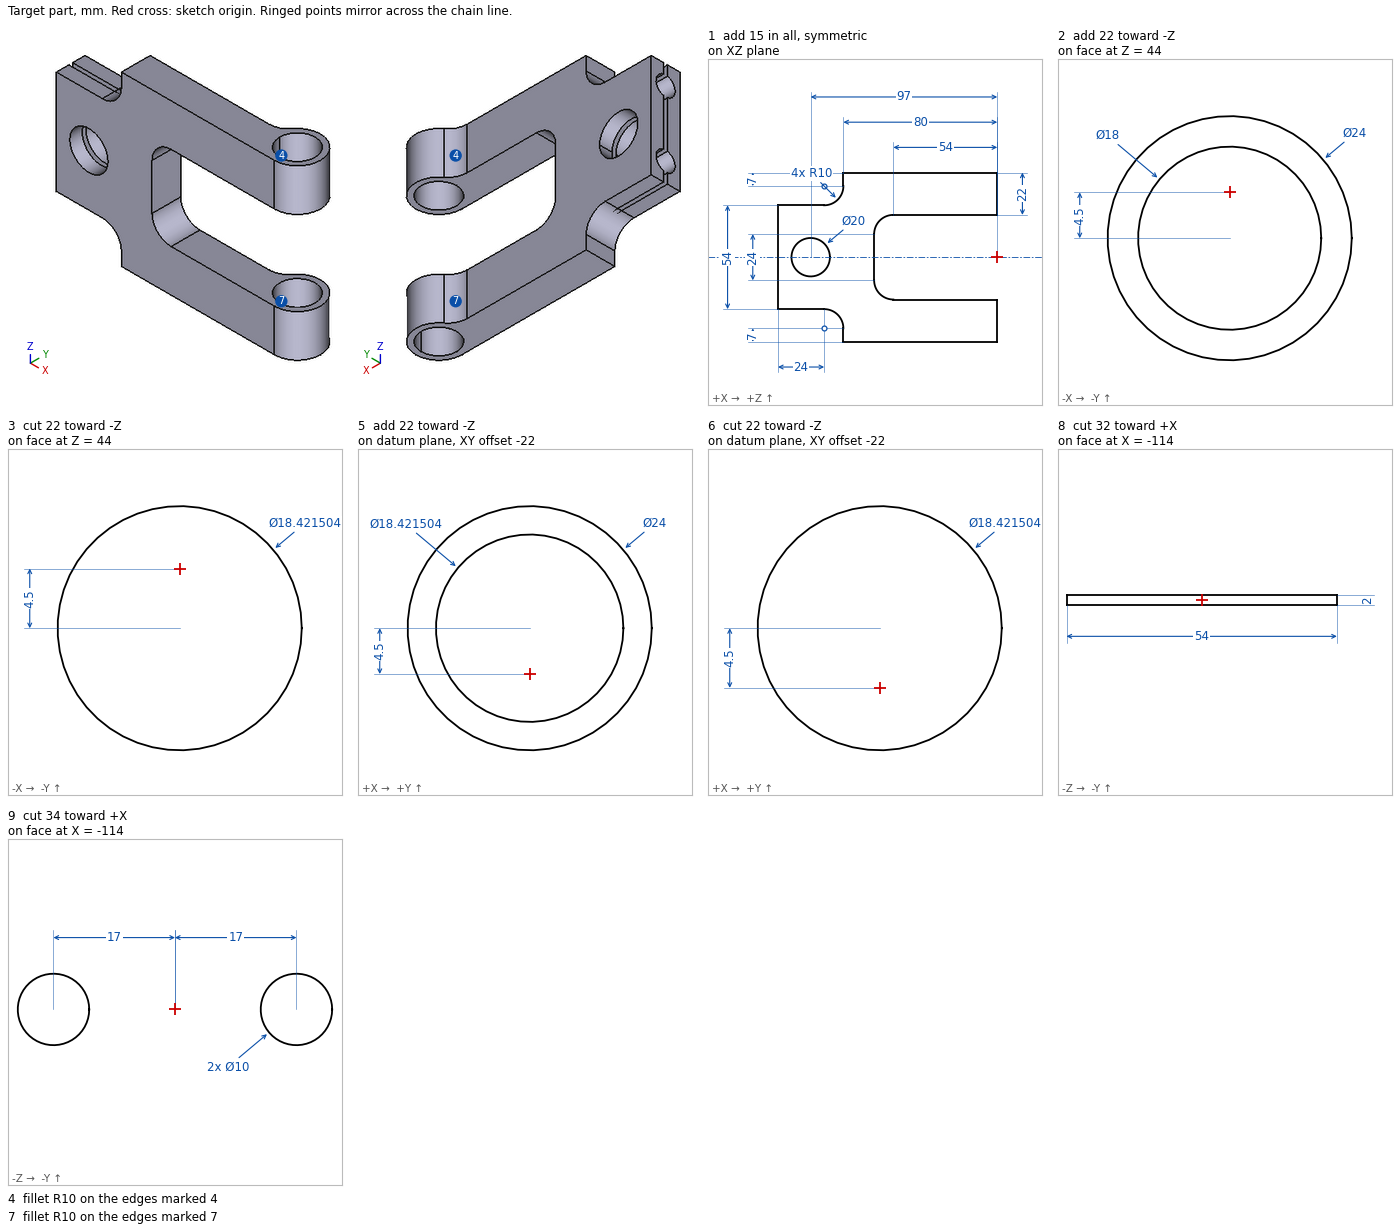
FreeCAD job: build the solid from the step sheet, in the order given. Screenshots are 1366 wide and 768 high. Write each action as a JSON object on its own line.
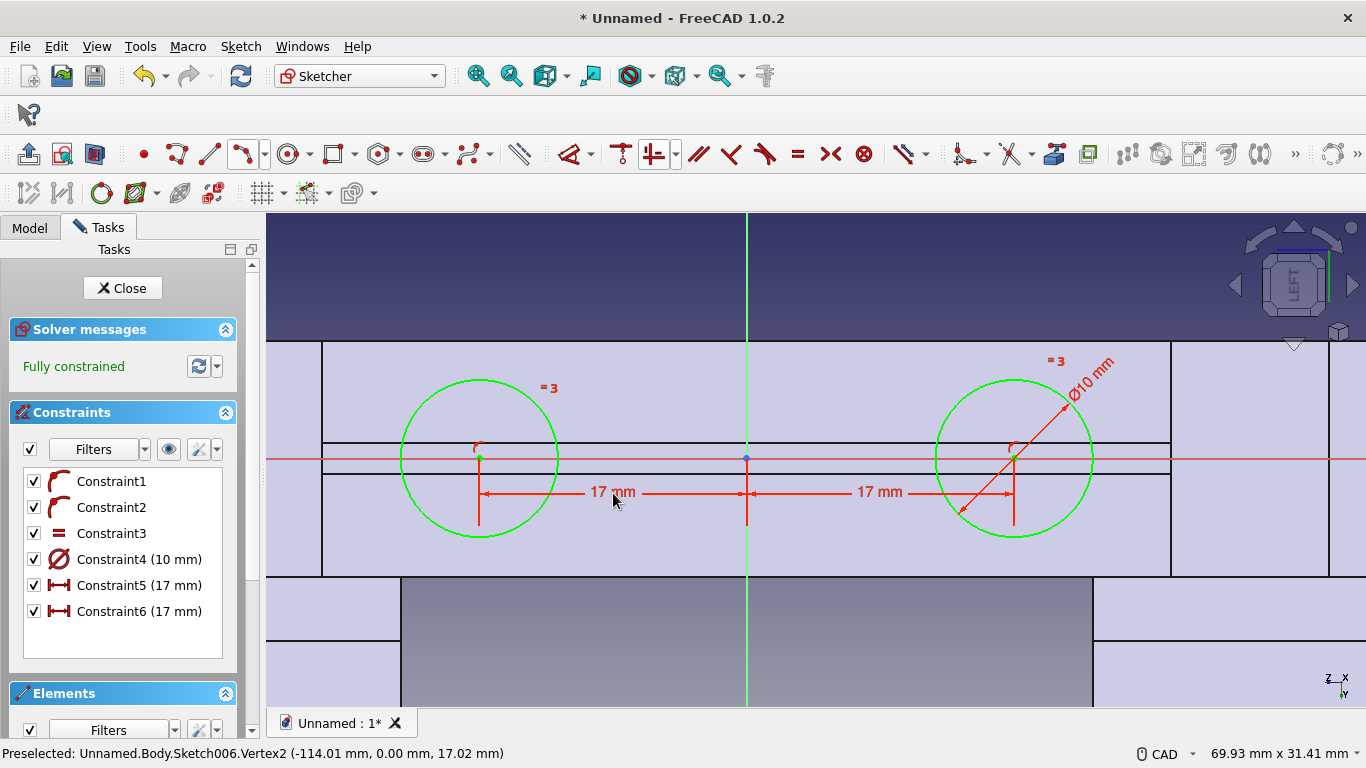
{"action": "left_click", "coordinate": [123, 288]}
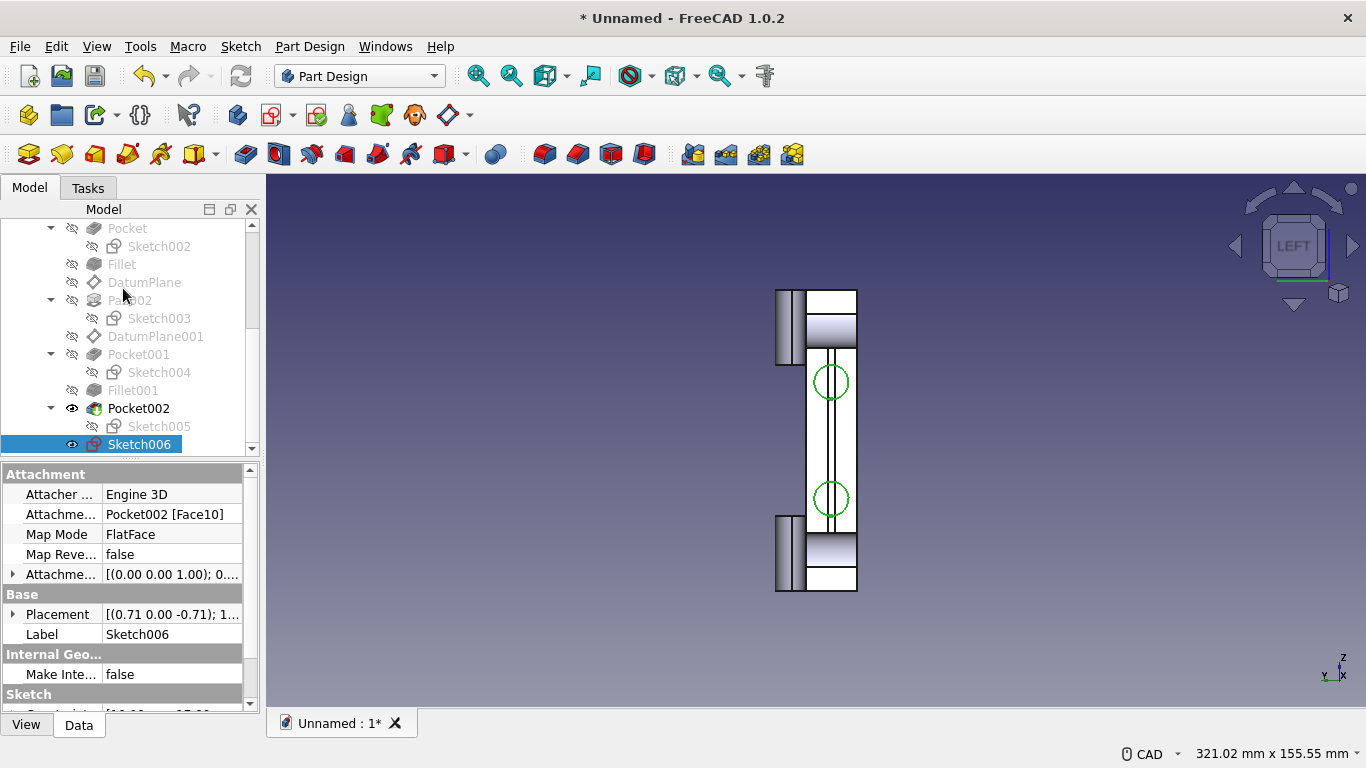
{"action": "left_click", "coordinate": [246, 154]}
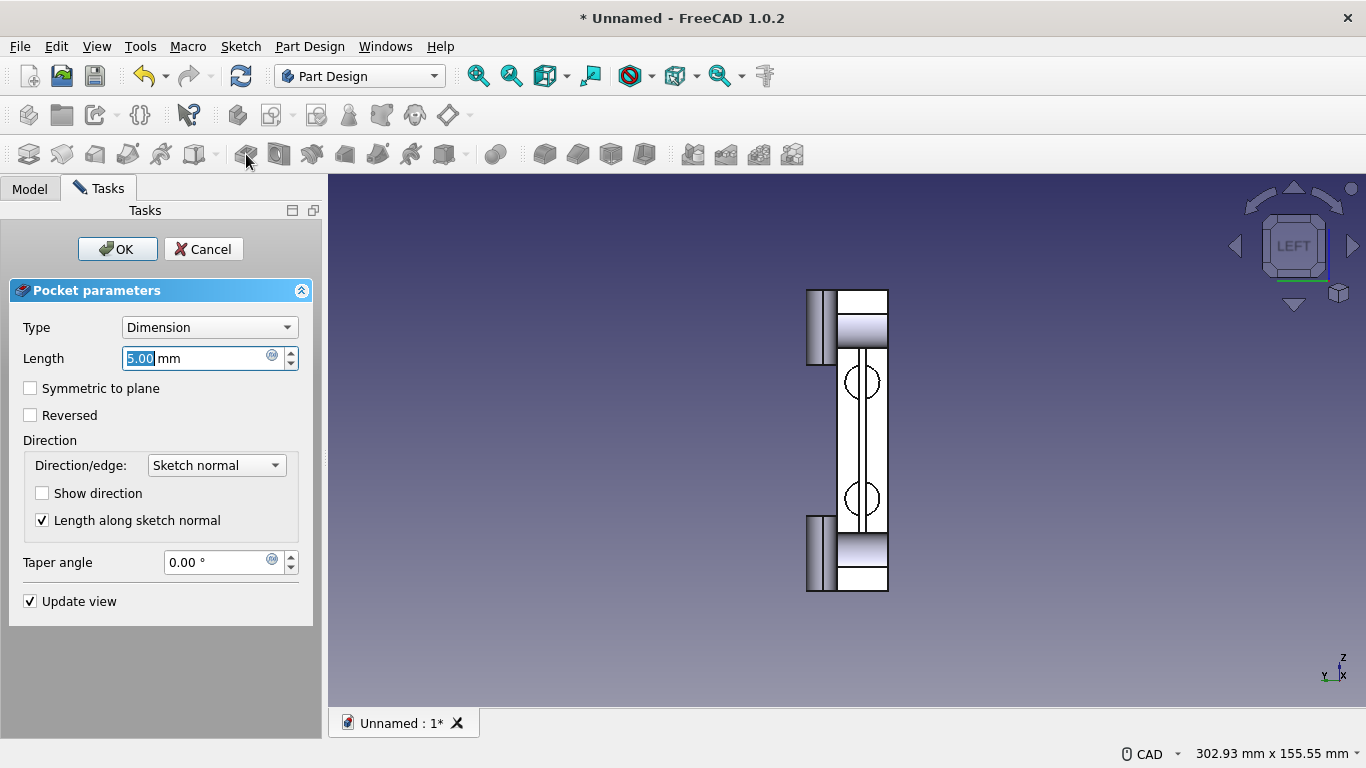
{"action": "type", "text": "34"}
{"action": "key", "text": "Tab"}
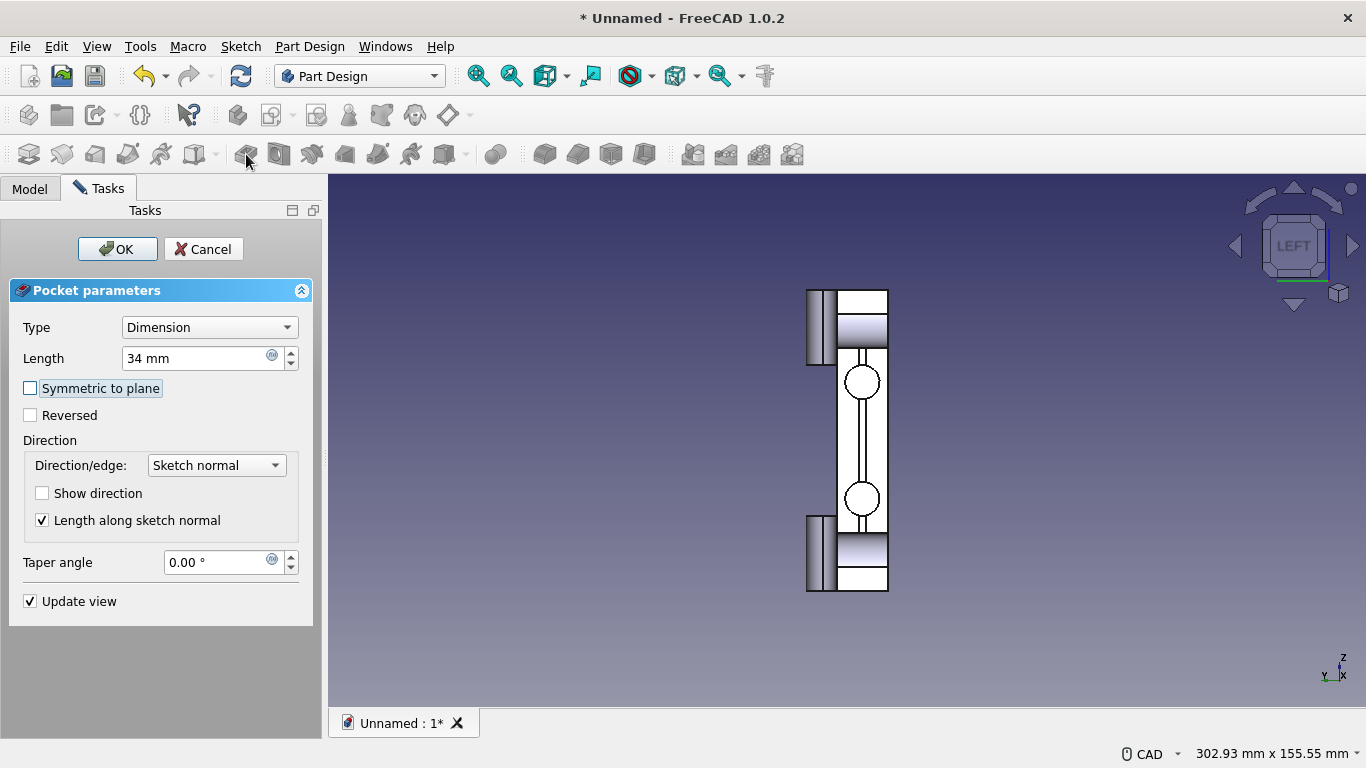
{"action": "left_click", "coordinate": [118, 249]}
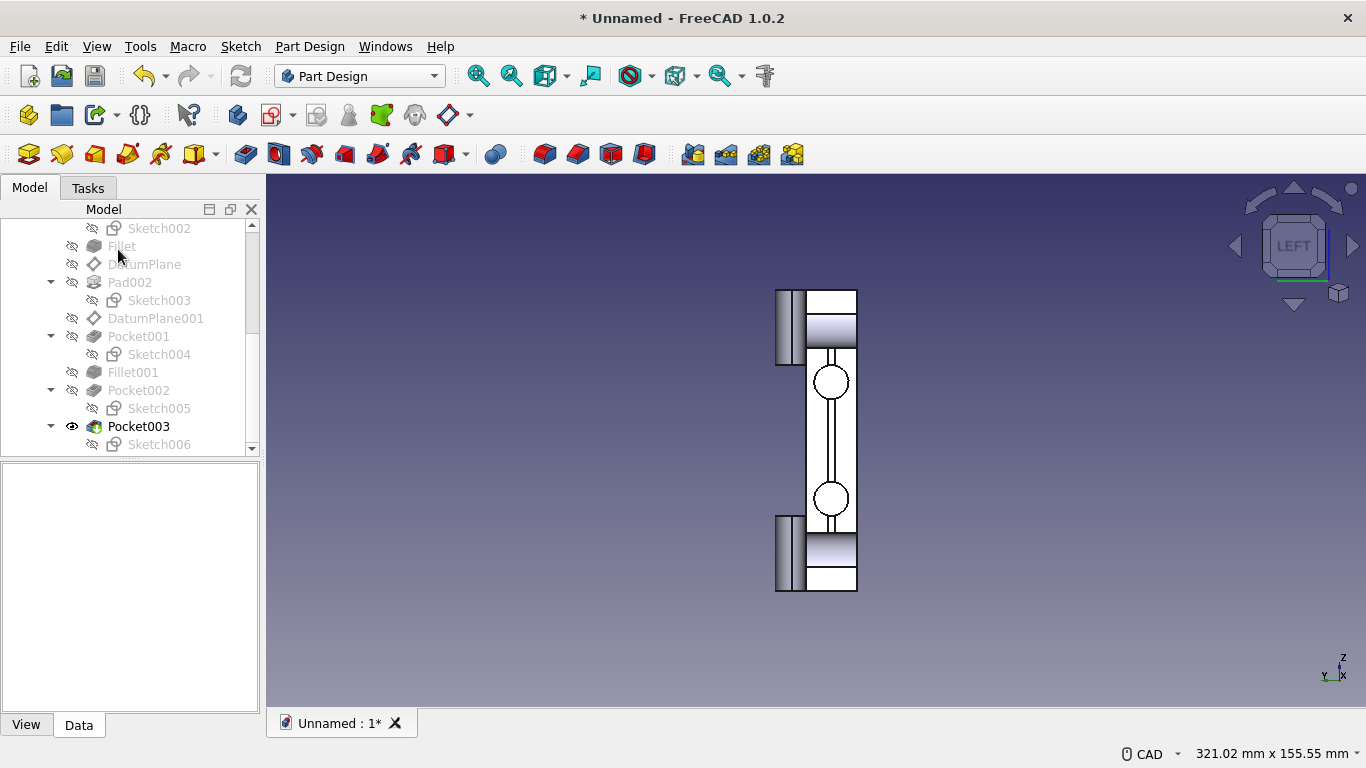
{"action": "key", "text": "0"}